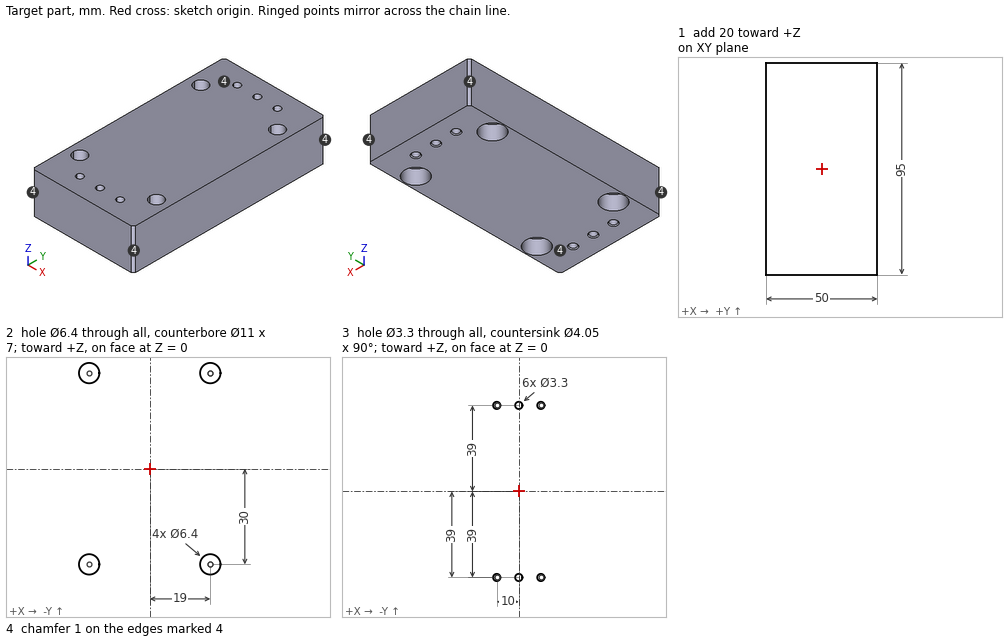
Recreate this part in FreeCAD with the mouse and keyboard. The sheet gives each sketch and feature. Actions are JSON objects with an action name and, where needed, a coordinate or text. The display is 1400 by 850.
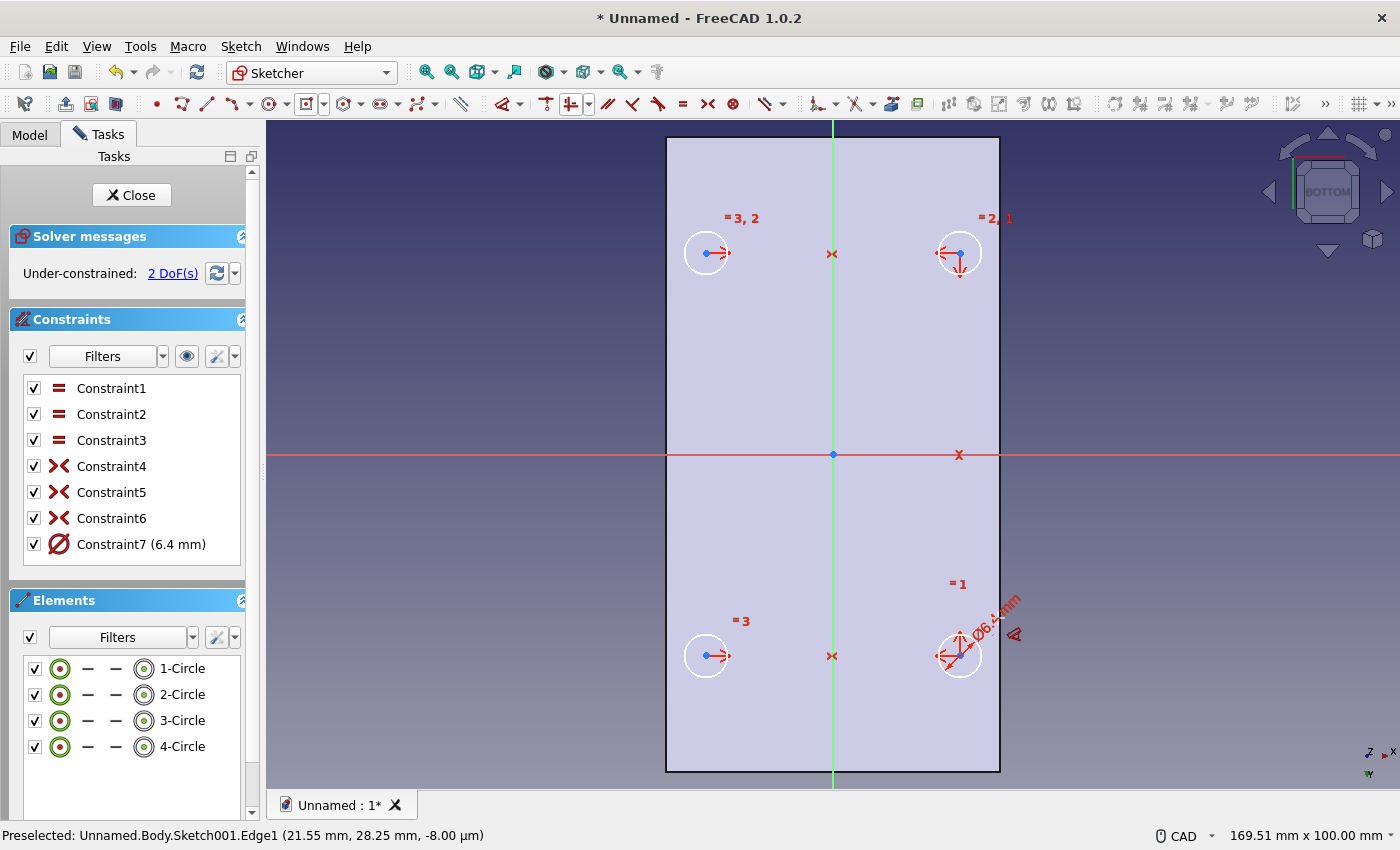
{"action": "left_click", "coordinate": [960, 656]}
{"action": "left_click", "coordinate": [896, 690]}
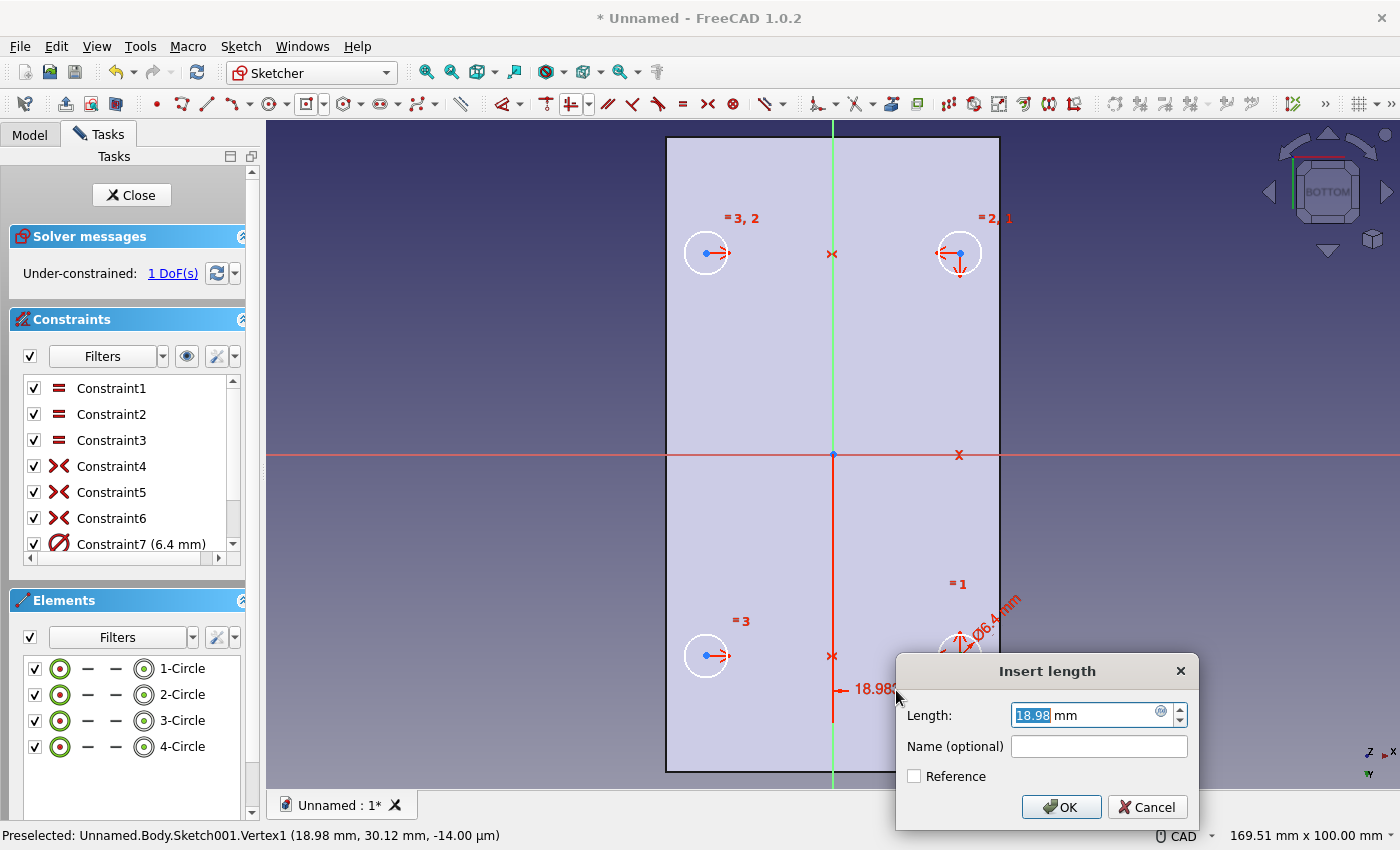
{"action": "type", "text": "19"}
{"action": "key", "text": "Return"}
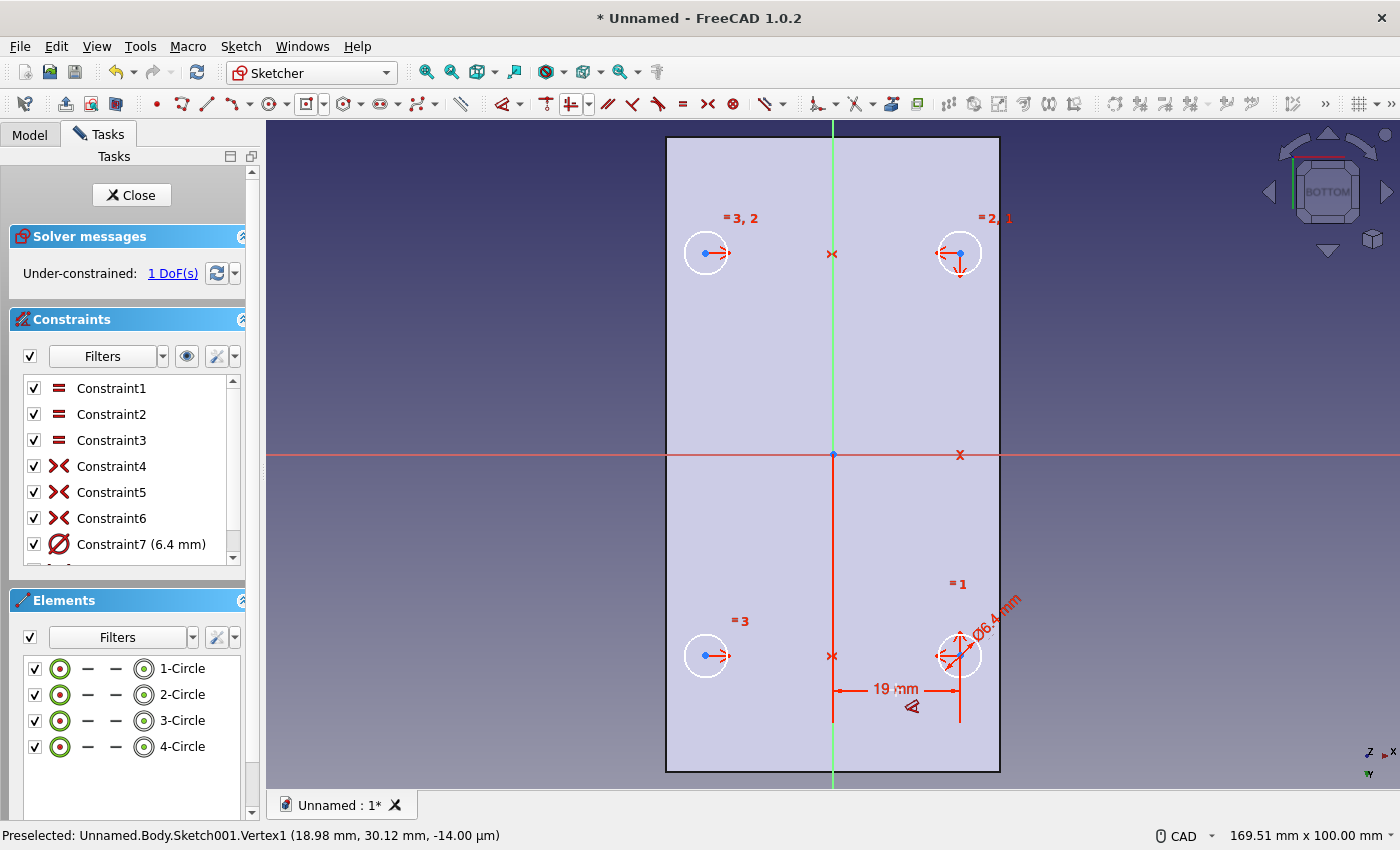
{"action": "left_click", "coordinate": [960, 656]}
{"action": "left_click", "coordinate": [994, 555]}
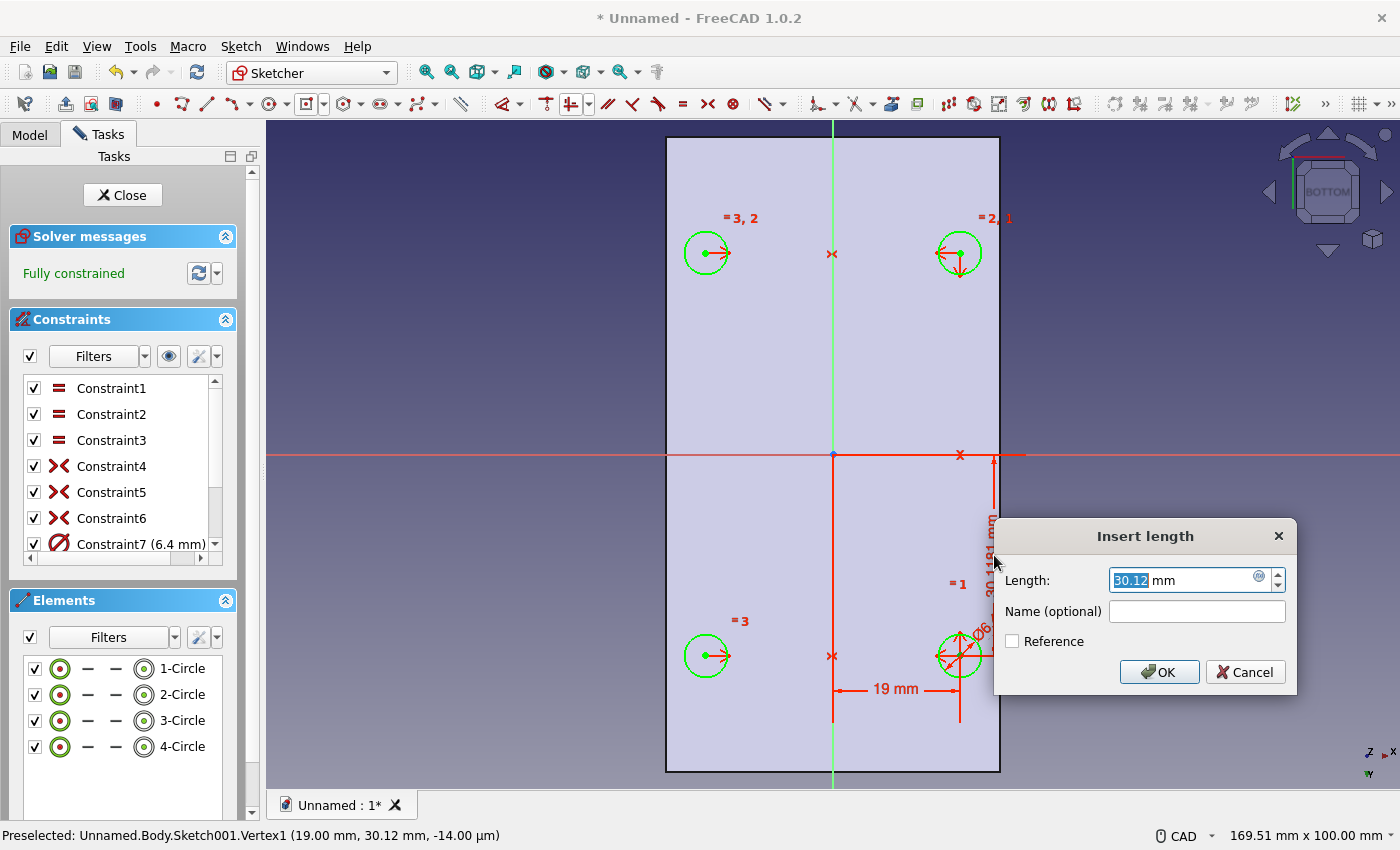
{"action": "type", "text": "30"}
{"action": "key", "text": "Return"}
{"action": "key", "text": "Escape"}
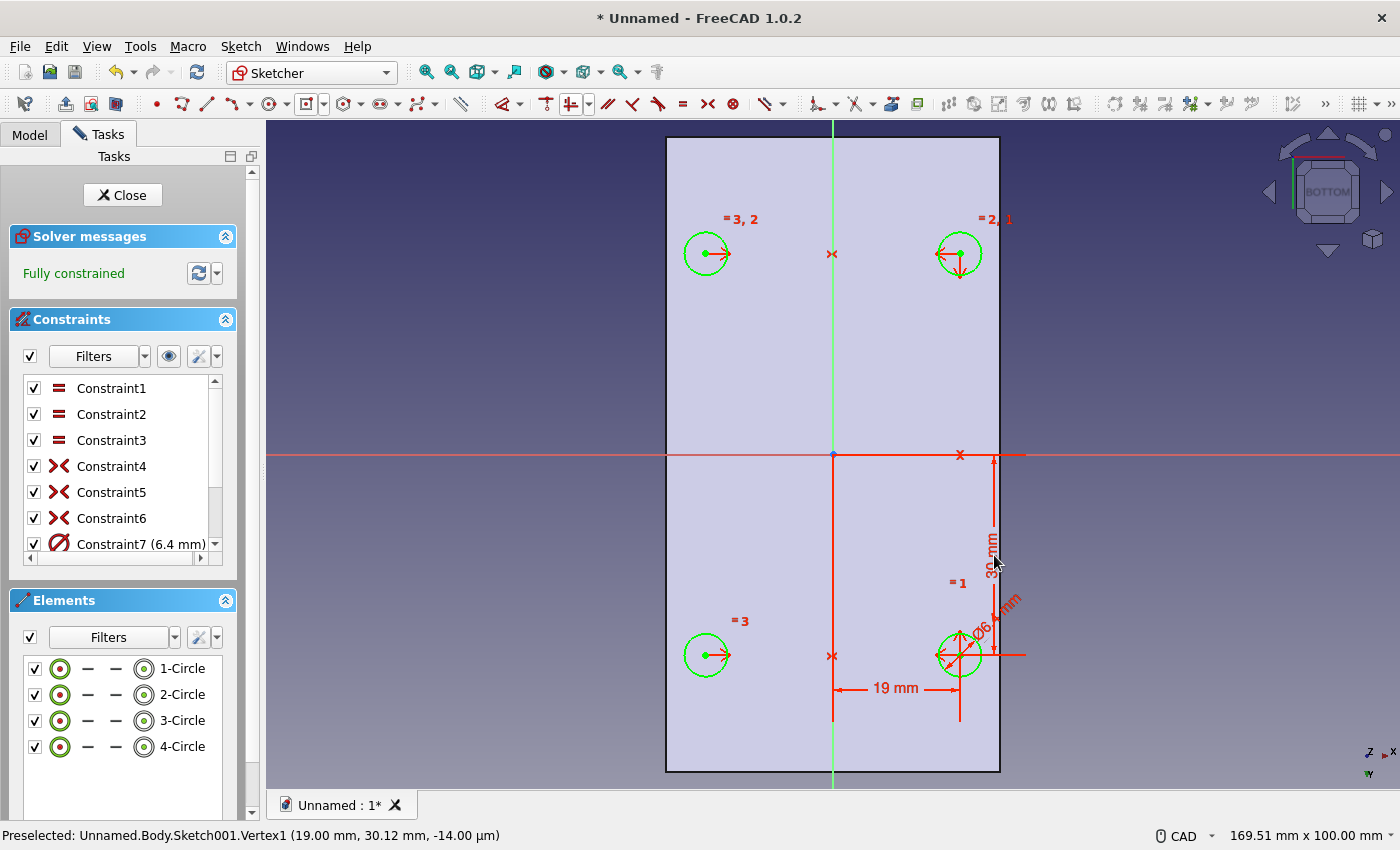
{"action": "left_click", "coordinate": [123, 195]}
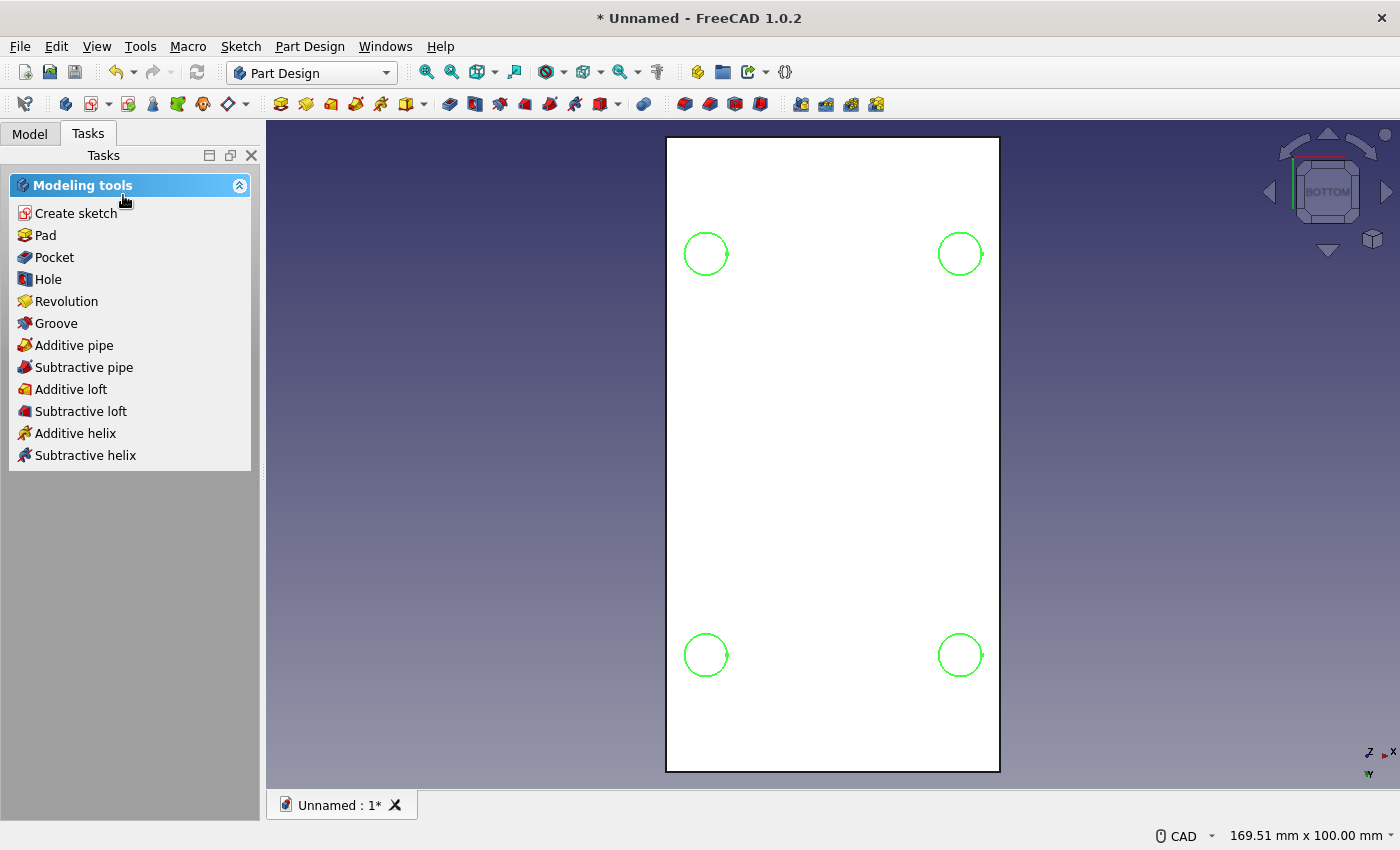
{"action": "left_click", "coordinate": [475, 104]}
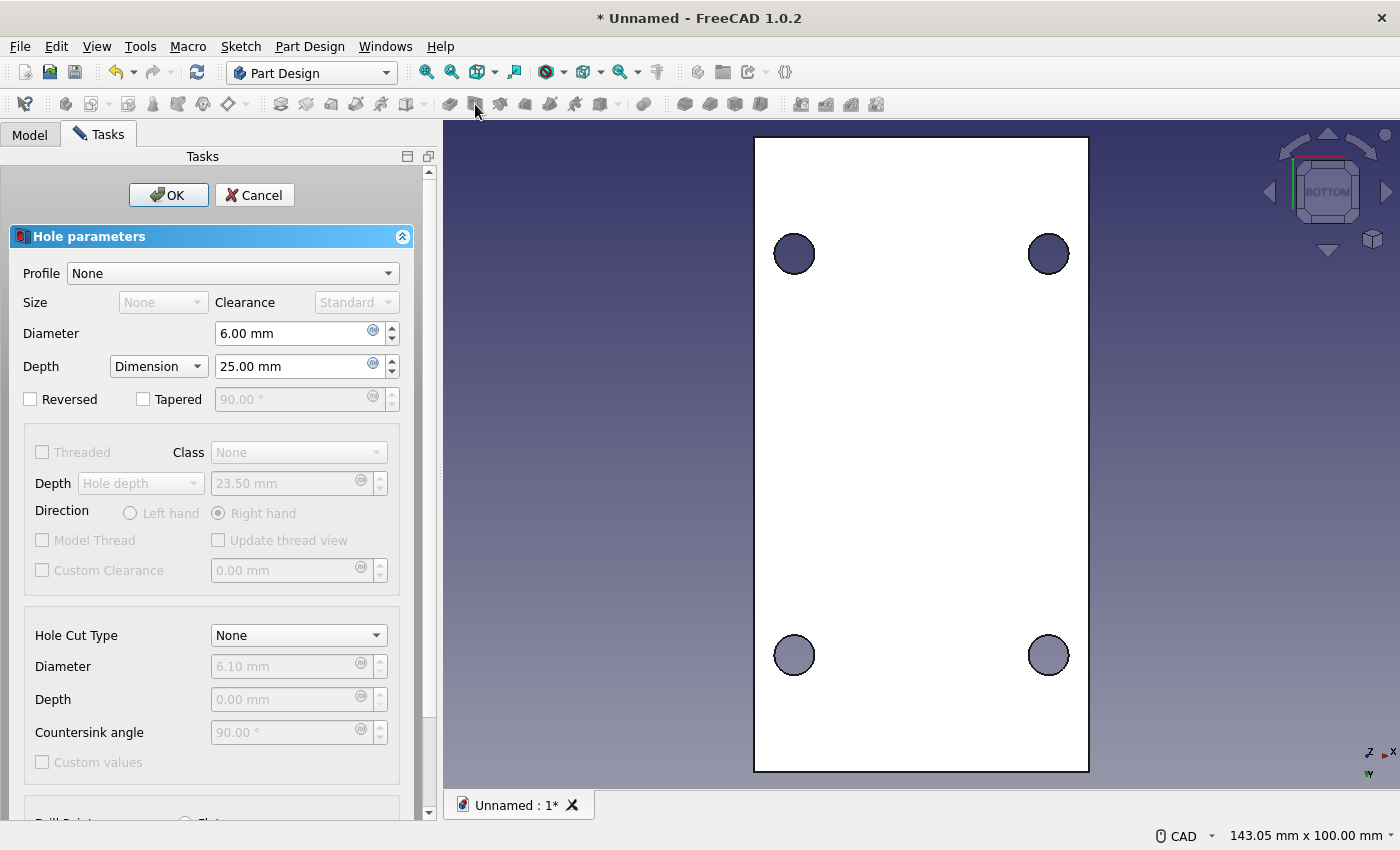
{"action": "triple_click", "coordinate": [300, 334]}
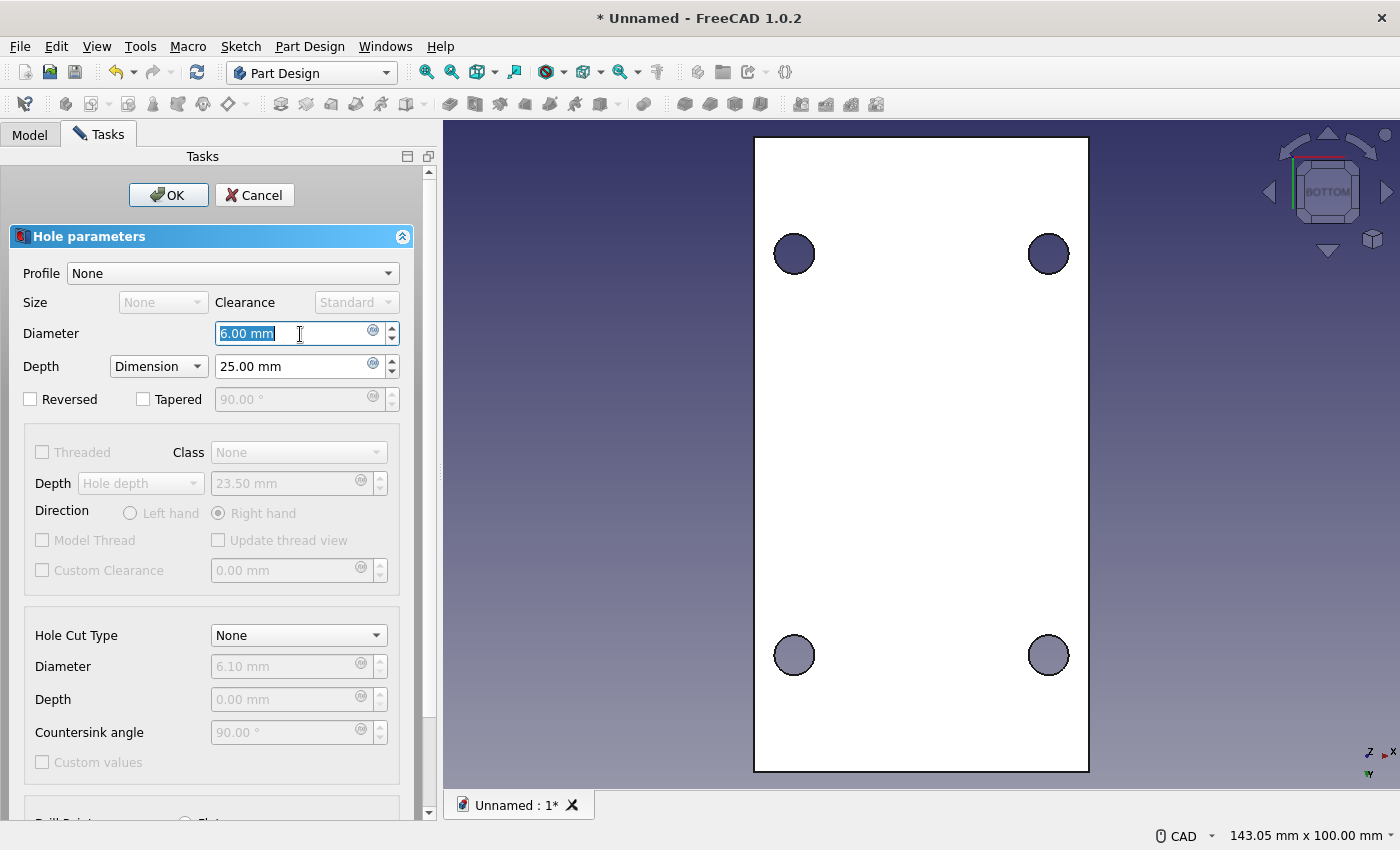
{"action": "type", "text": "6.4"}
{"action": "key", "text": "Tab"}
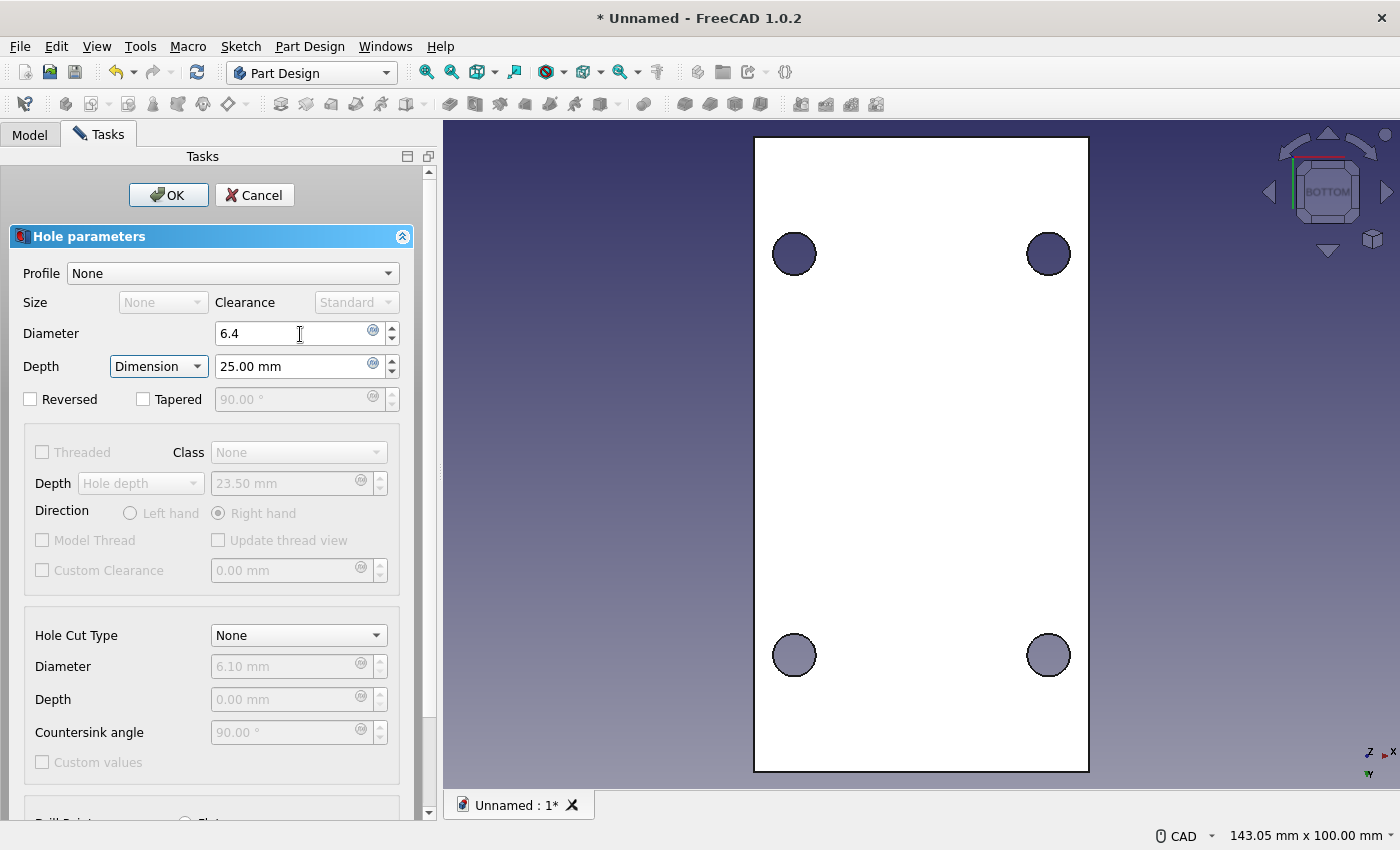
{"action": "left_click", "coordinate": [160, 366]}